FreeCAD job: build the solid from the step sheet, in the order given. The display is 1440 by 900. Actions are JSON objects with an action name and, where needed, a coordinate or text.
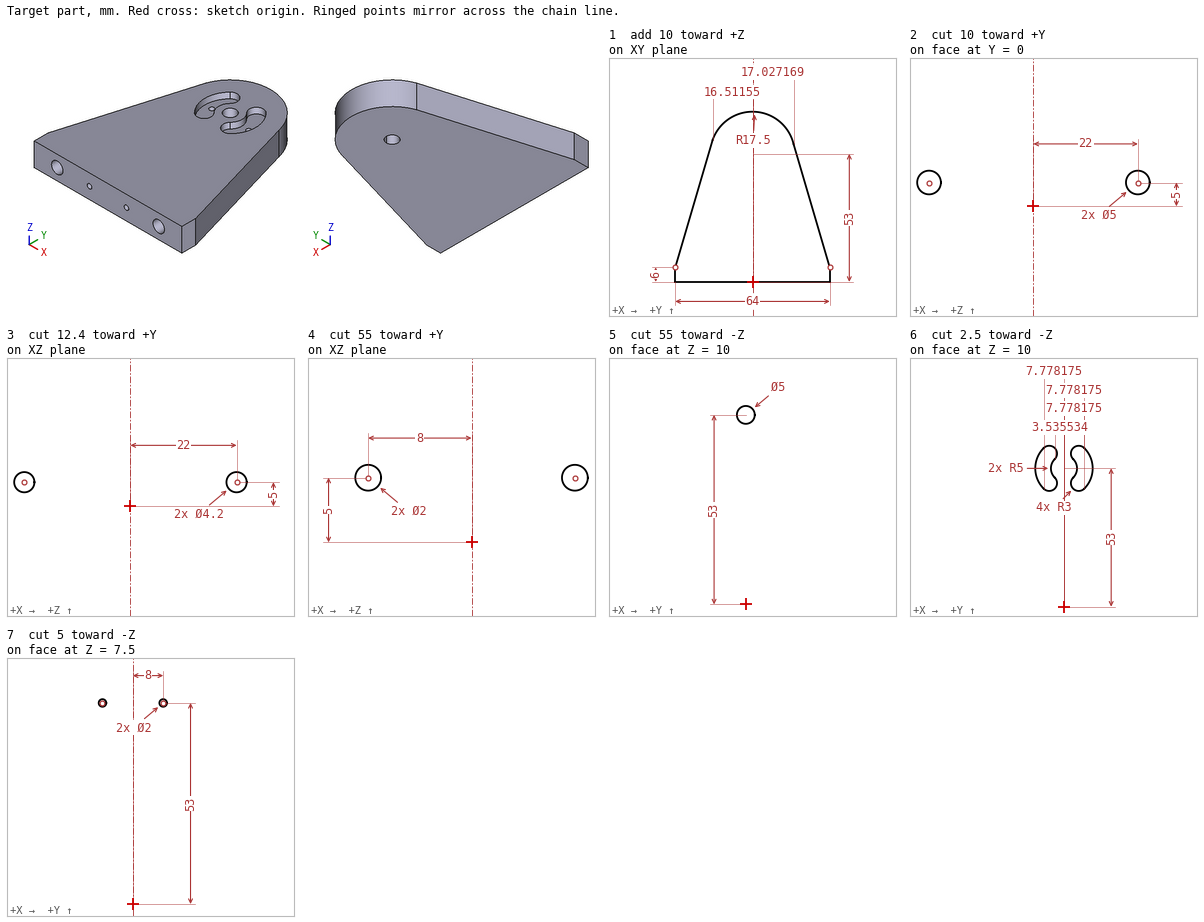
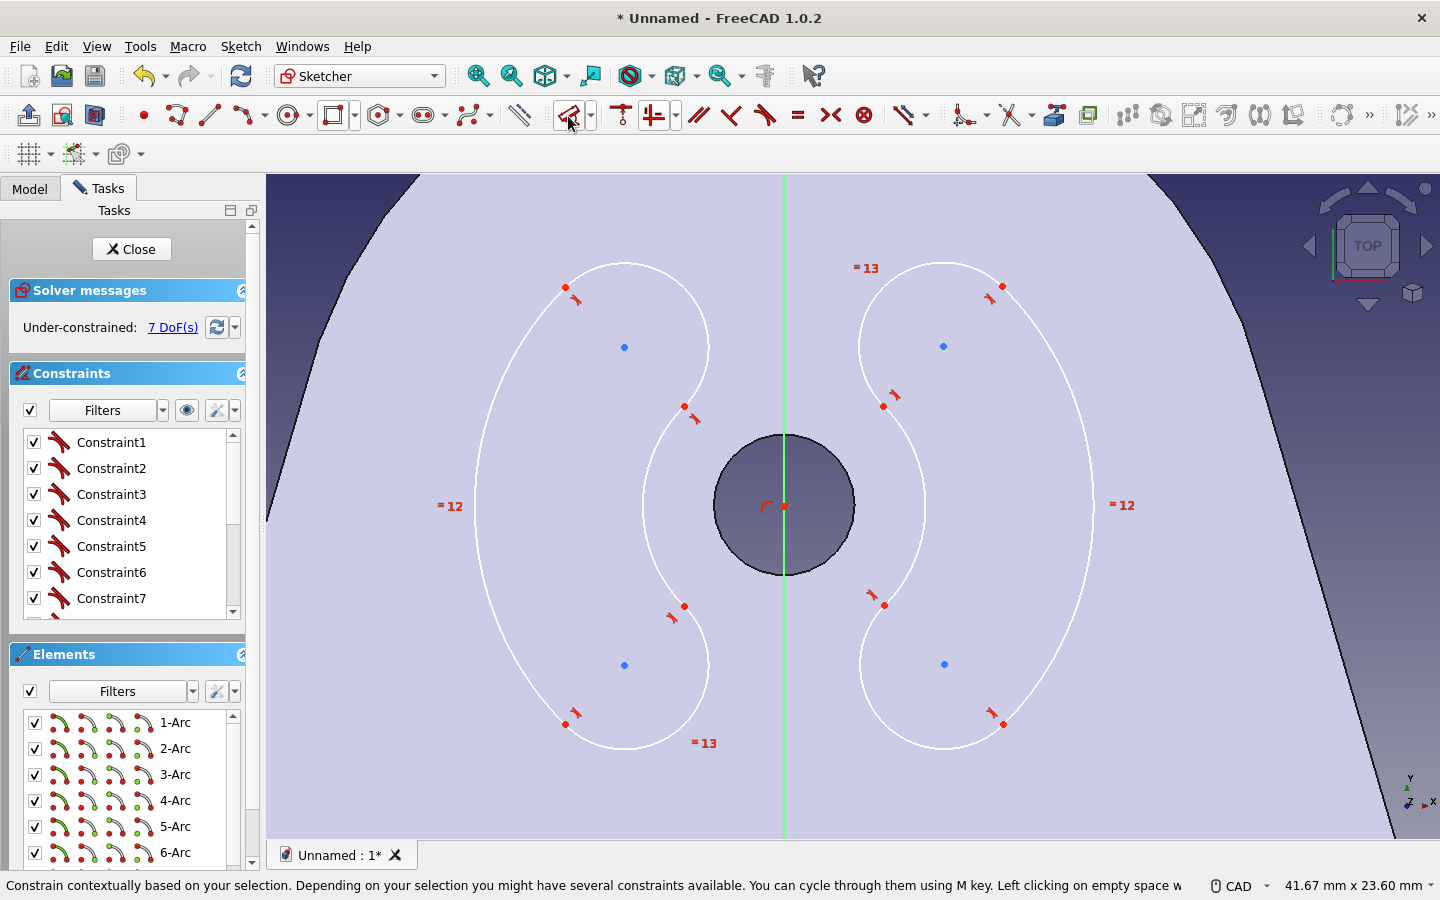
{"action": "left_click", "coordinate": [638, 748]}
{"action": "left_click", "coordinate": [643, 780]}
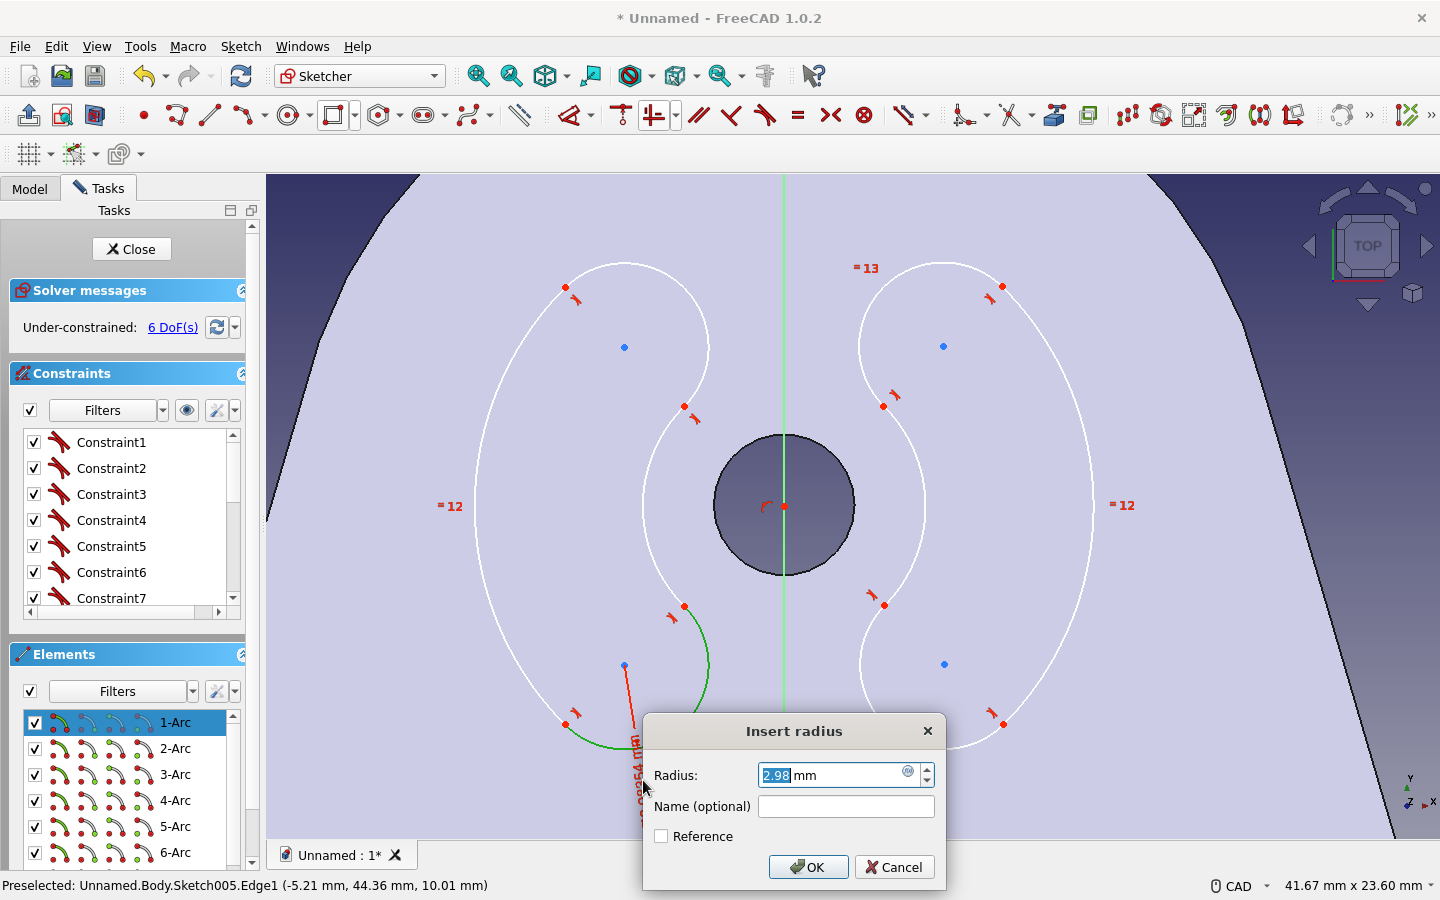
{"action": "type", "text": "3"}
{"action": "key", "text": "Return"}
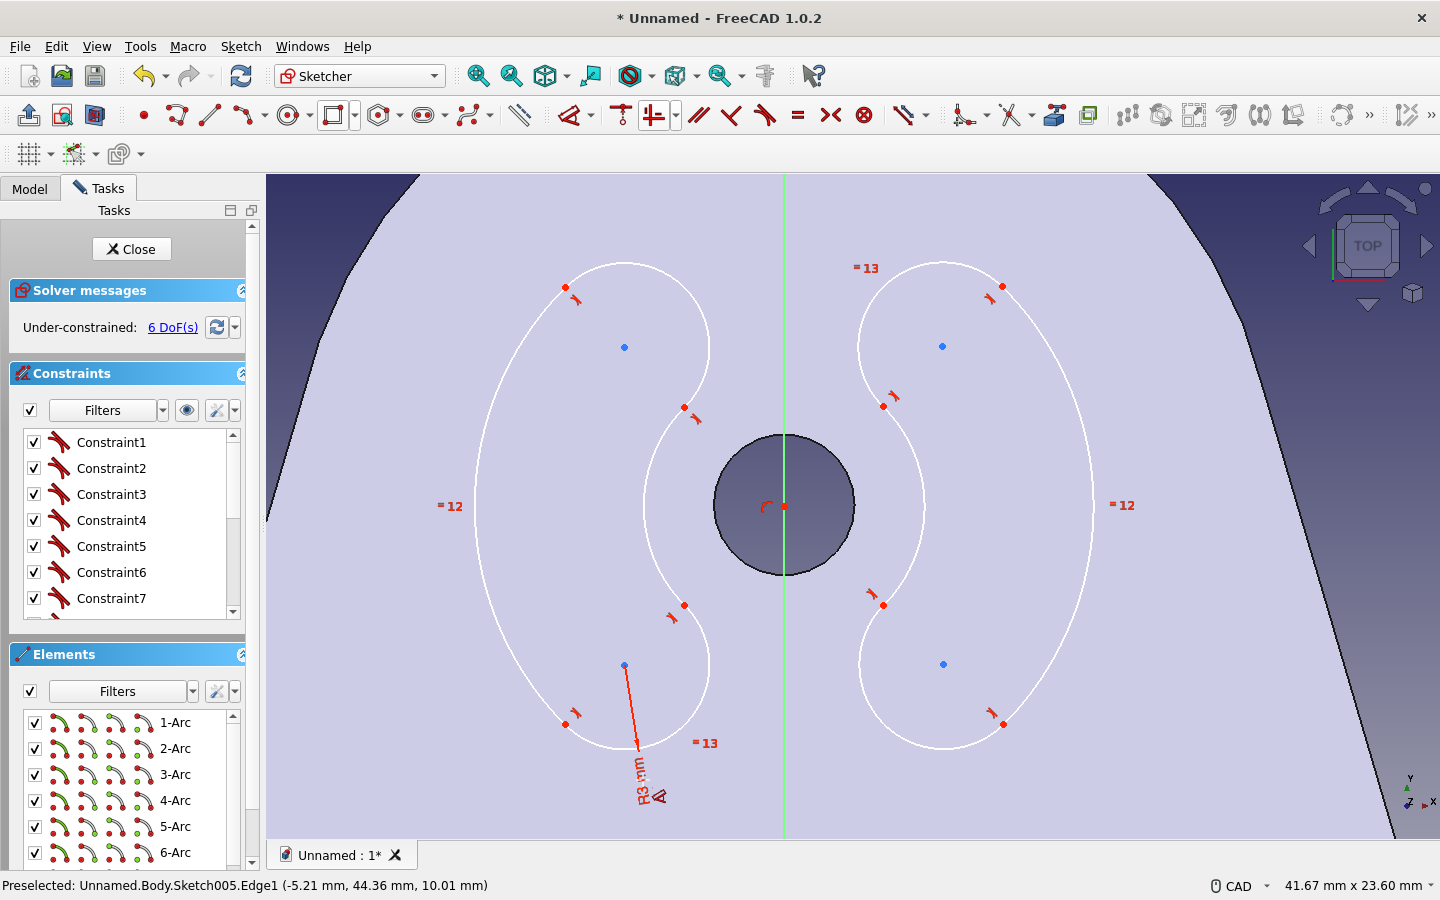
{"action": "left_click", "coordinate": [651, 463]}
{"action": "left_click", "coordinate": [621, 453]}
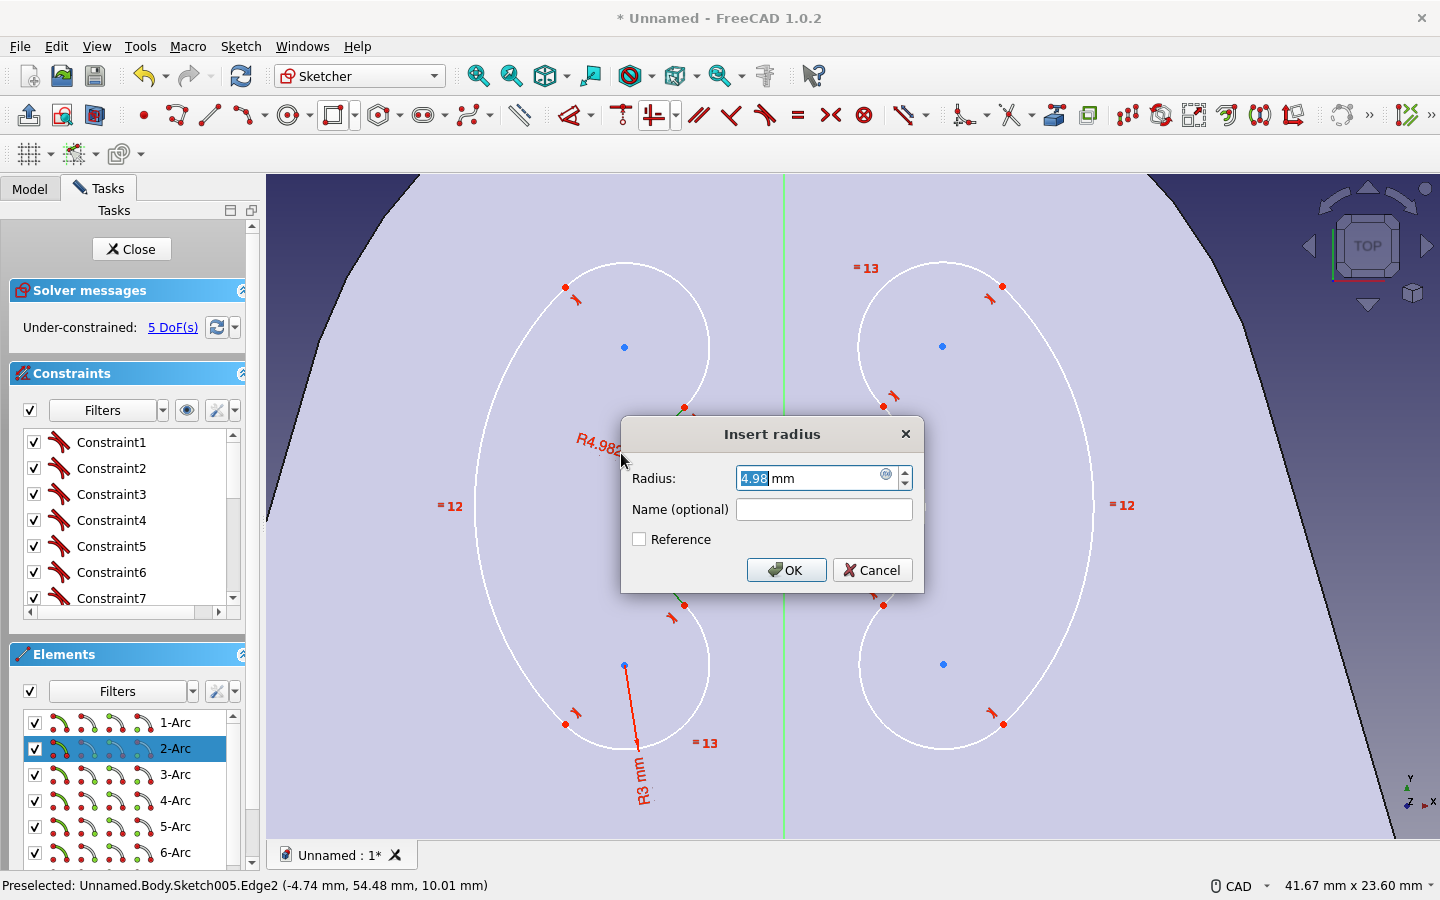
{"action": "type", "text": "5"}
{"action": "key", "text": "Return"}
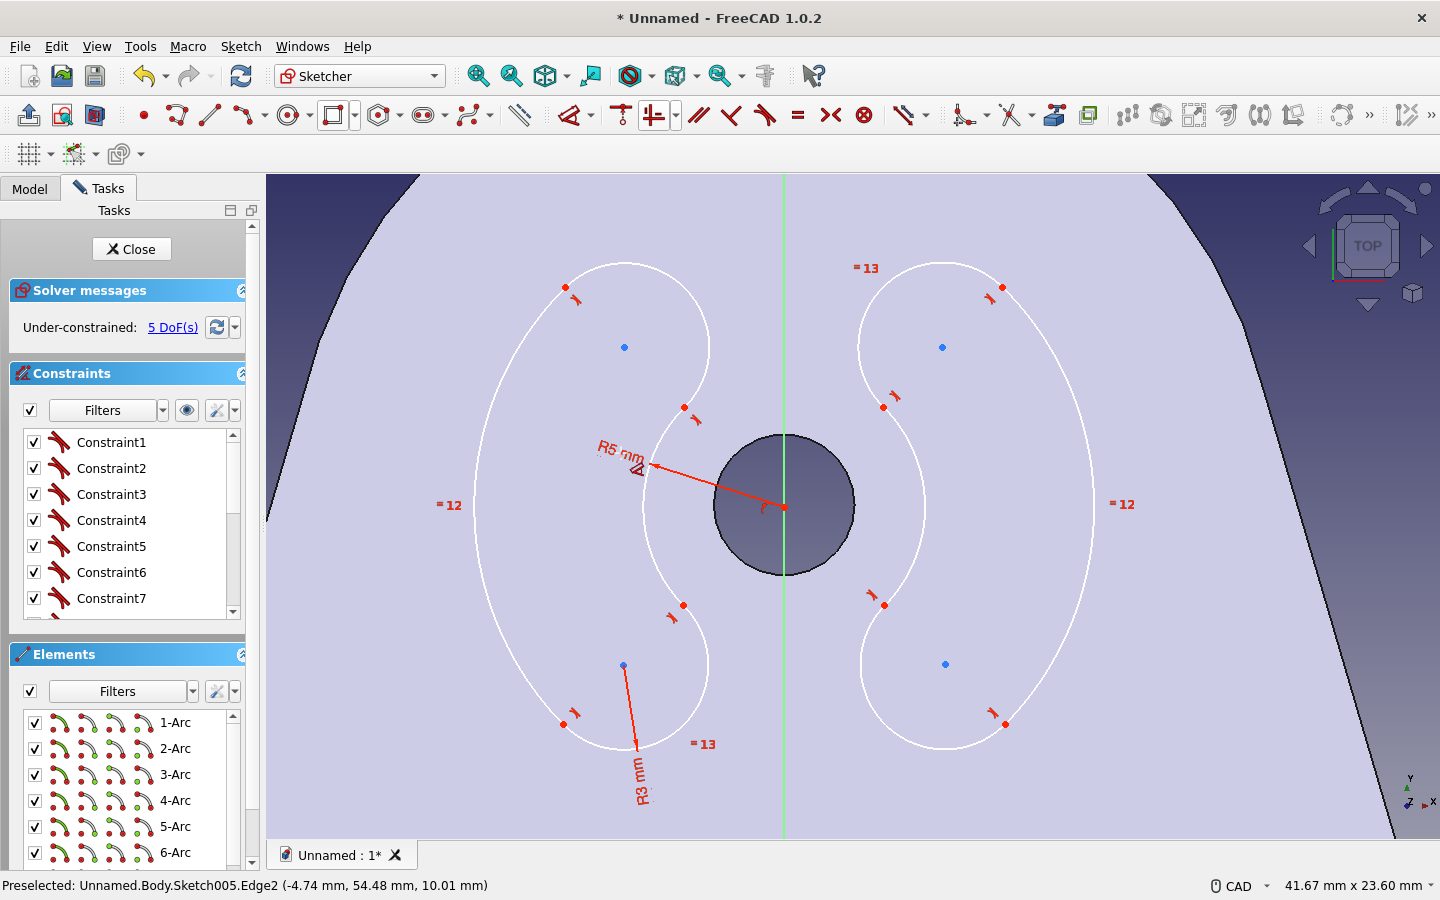
{"action": "left_click", "coordinate": [784, 507]}
{"action": "left_click", "coordinate": [818, 659]}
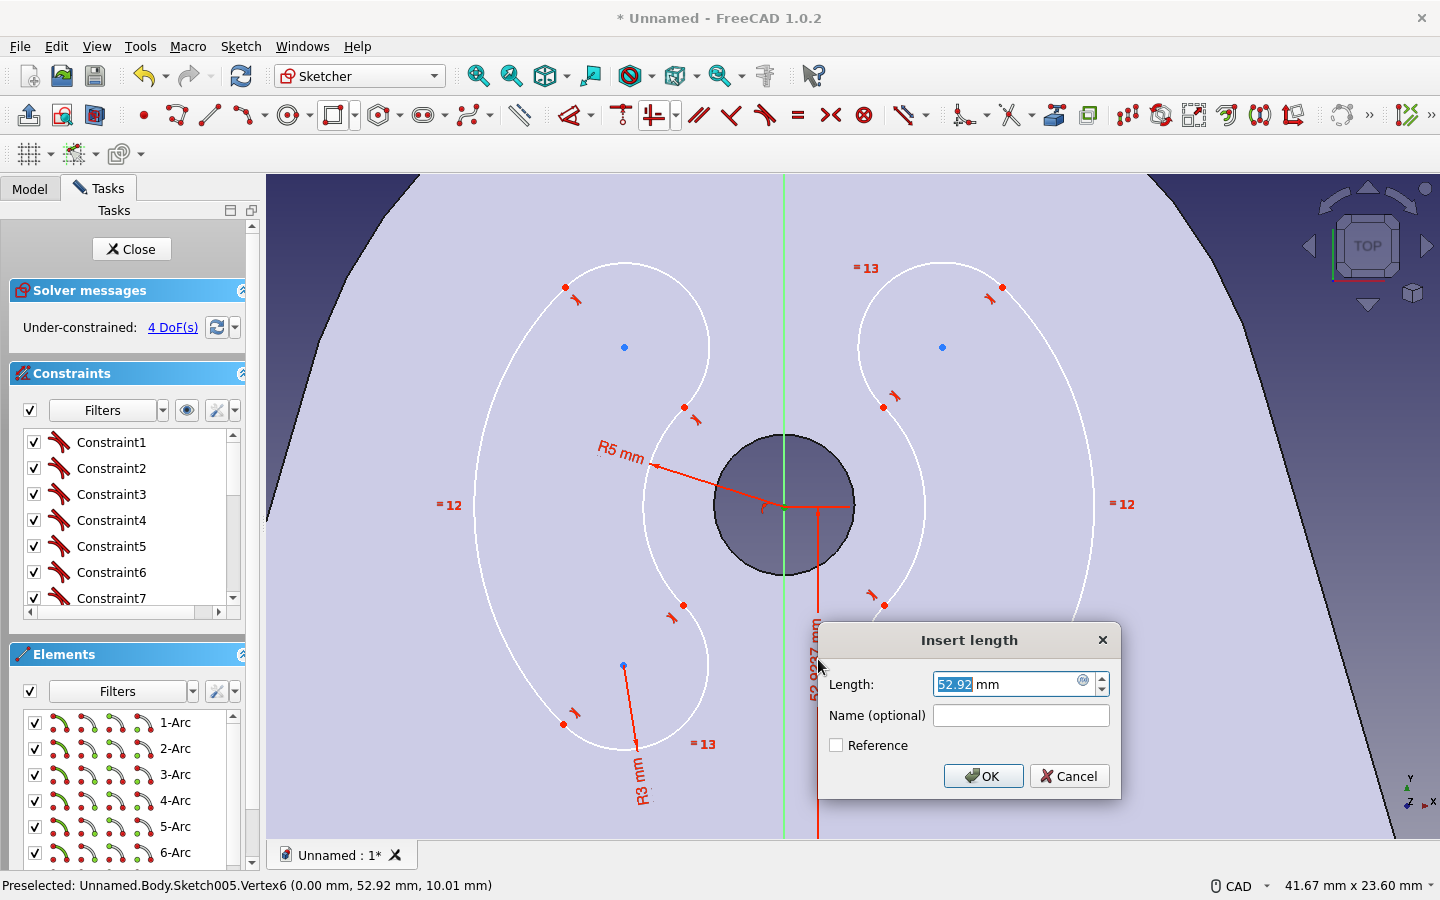
{"action": "type", "text": "53"}
{"action": "key", "text": "Return"}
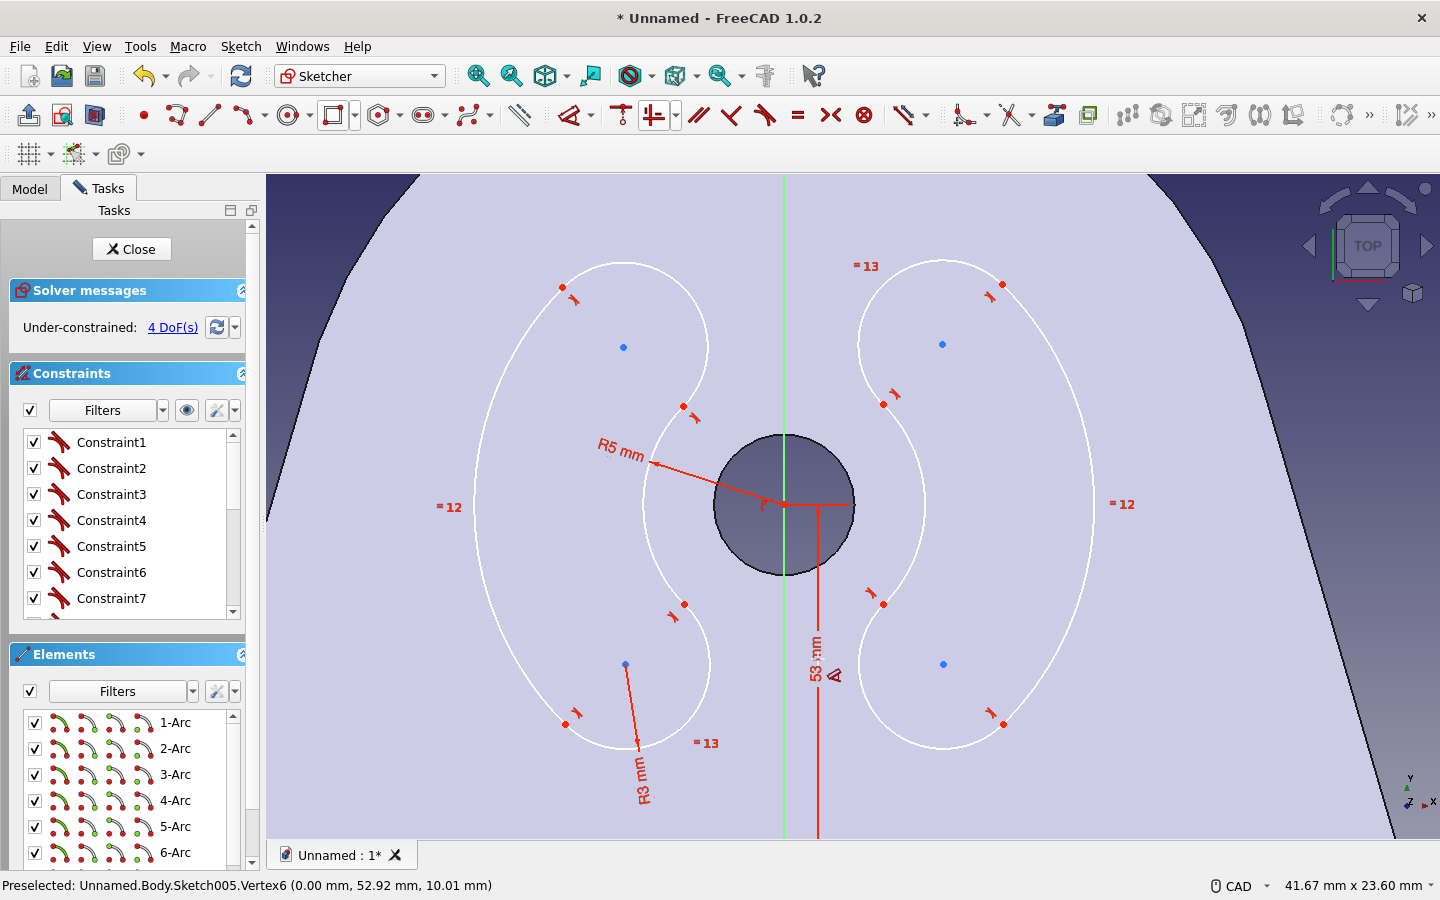
{"action": "left_click", "coordinate": [566, 725]}
{"action": "left_click", "coordinate": [675, 691]}